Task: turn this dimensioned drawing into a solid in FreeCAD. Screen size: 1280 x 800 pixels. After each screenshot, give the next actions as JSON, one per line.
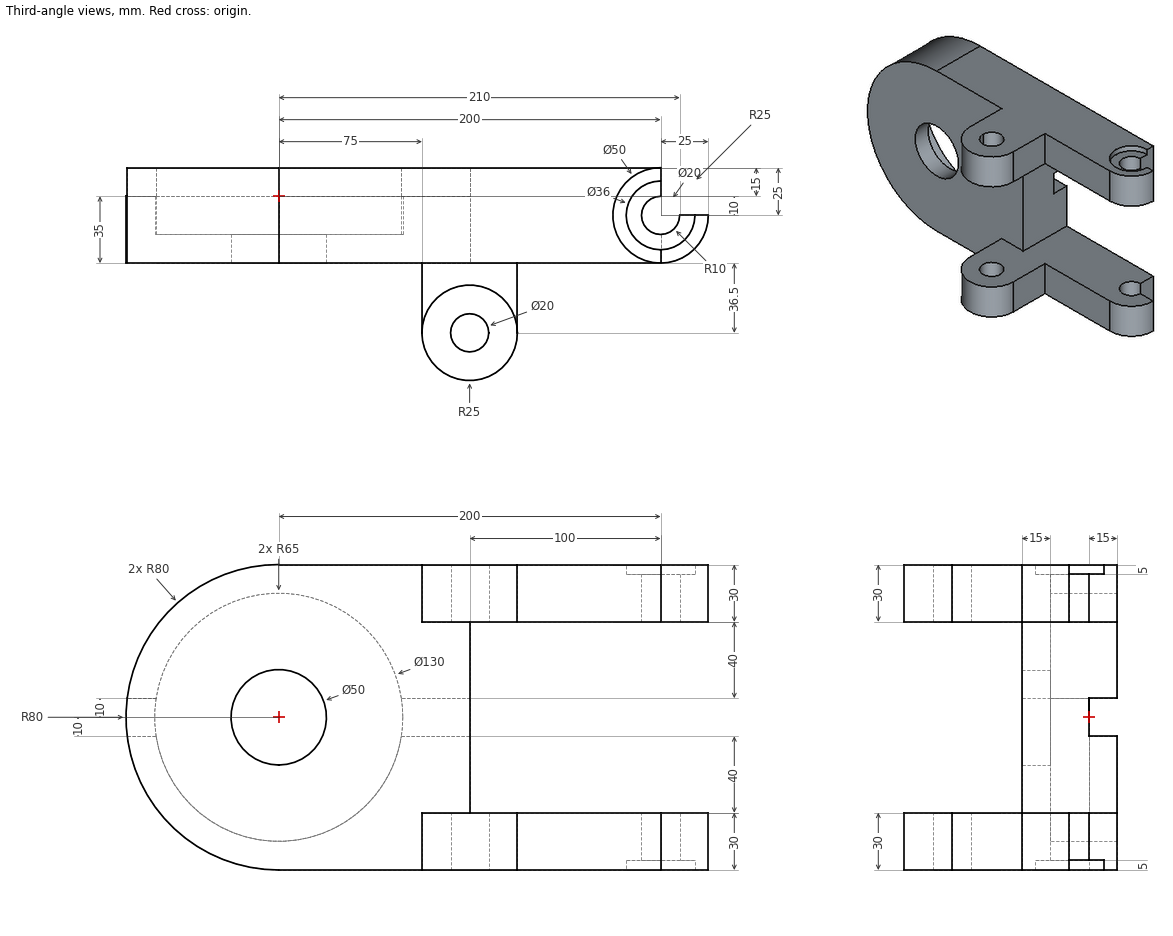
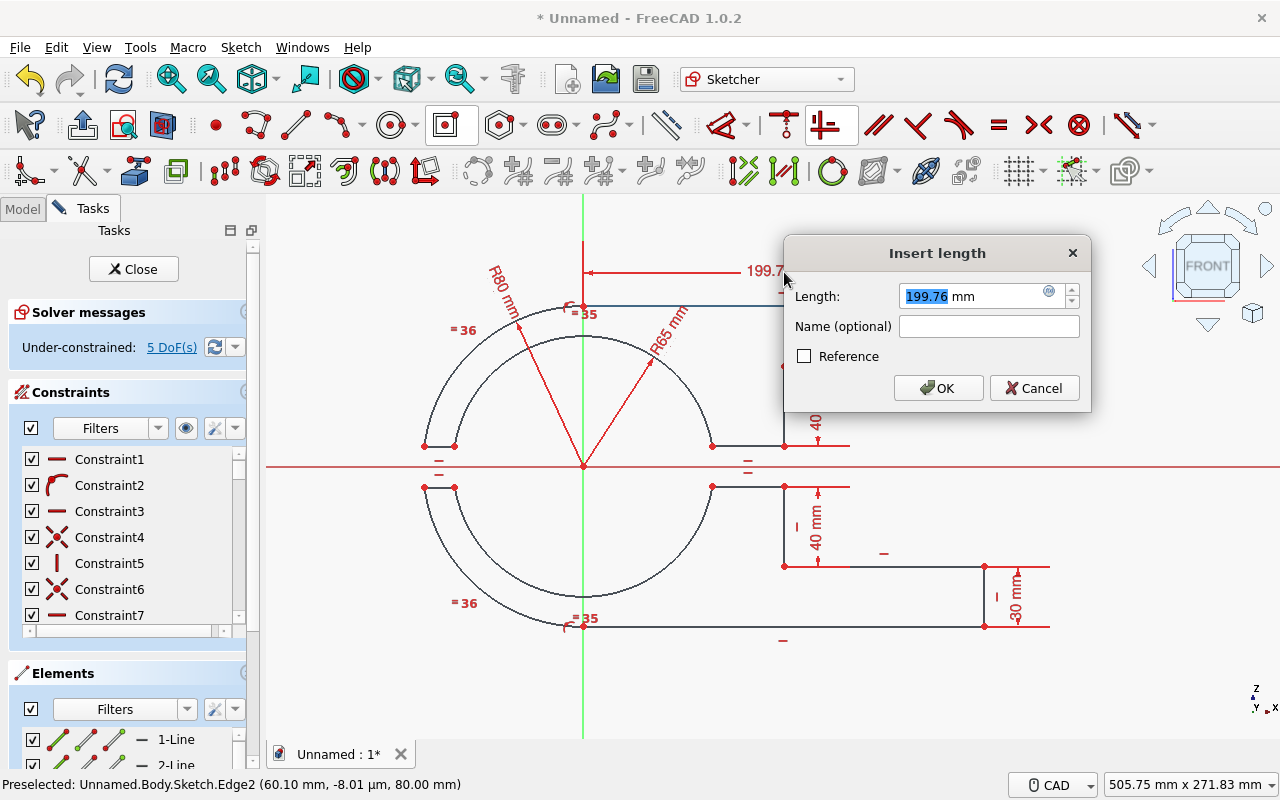
{"action": "type", "text": "200"}
{"action": "key", "text": "Return"}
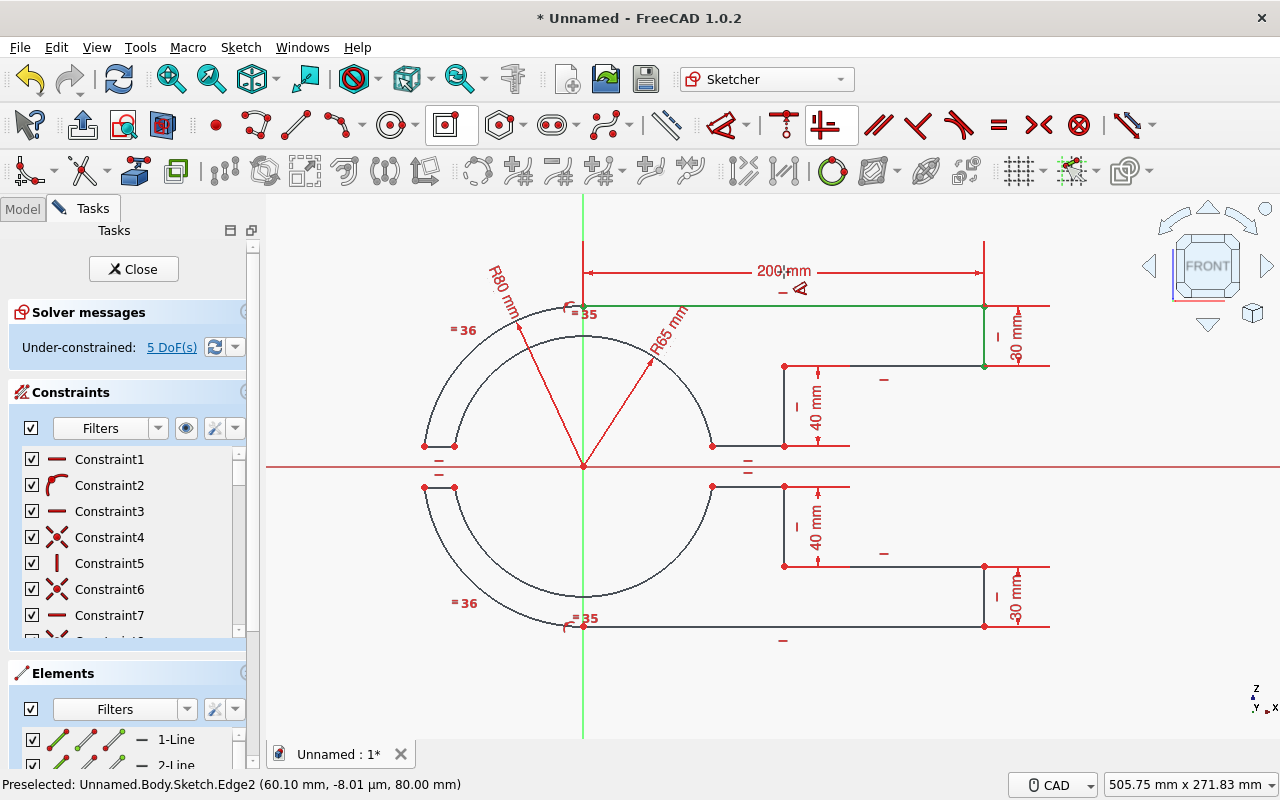
{"action": "left_click", "coordinate": [924, 366]}
{"action": "left_click", "coordinate": [884, 332]}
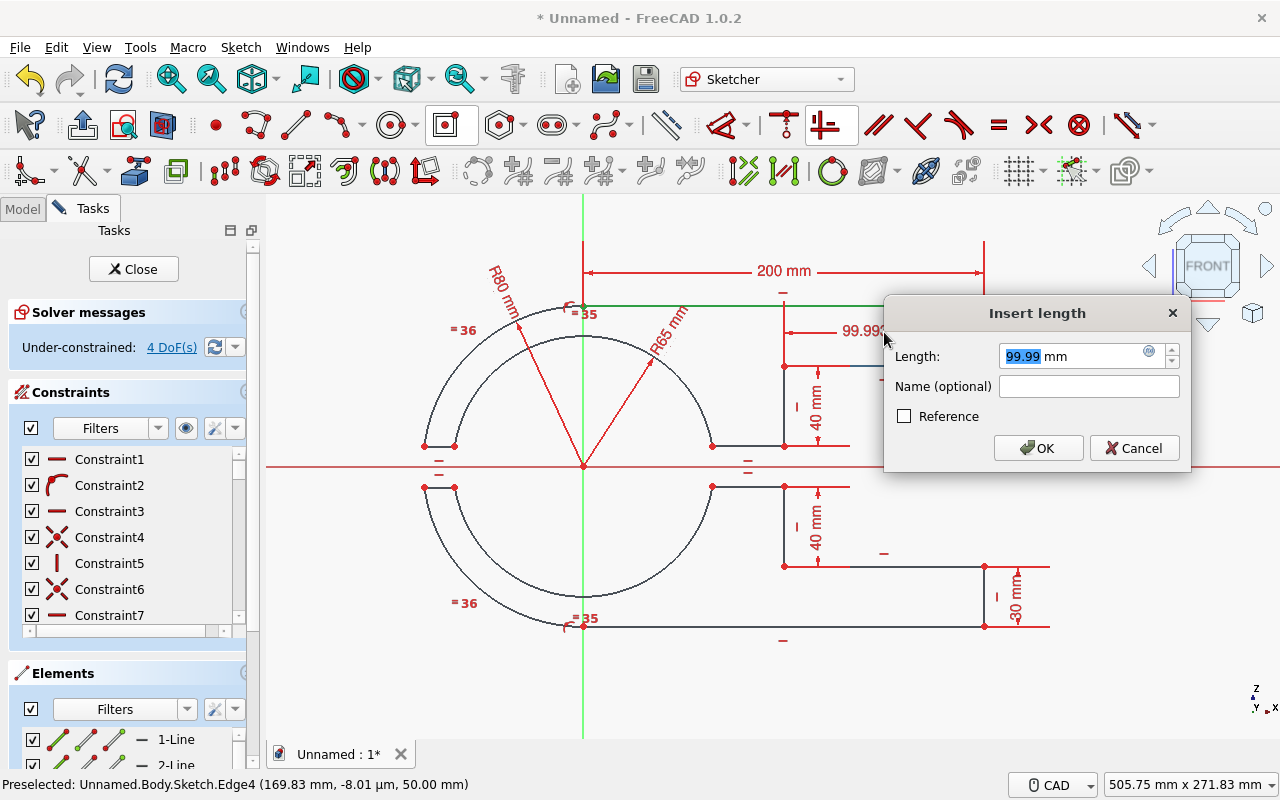
{"action": "type", "text": "100"}
{"action": "key", "text": "Return"}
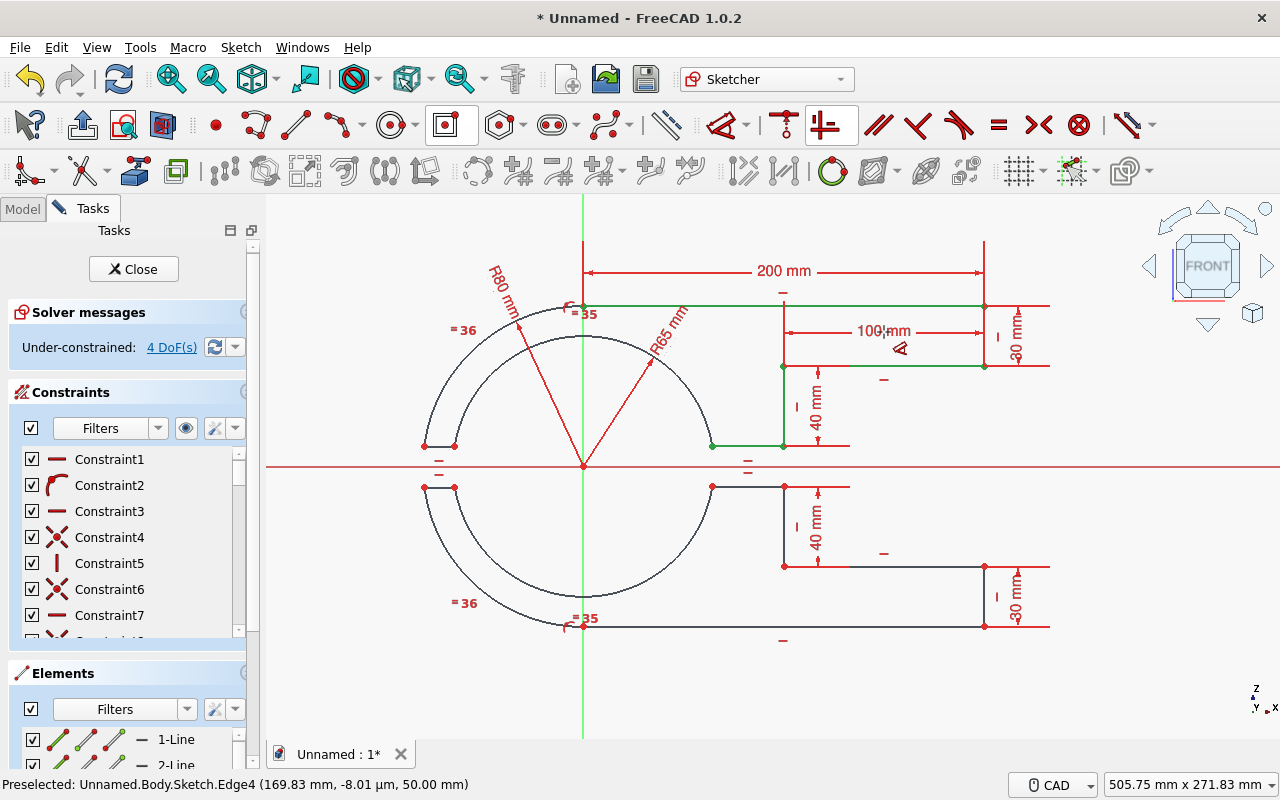
{"action": "left_click", "coordinate": [844, 567]}
{"action": "left_click", "coordinate": [884, 601]}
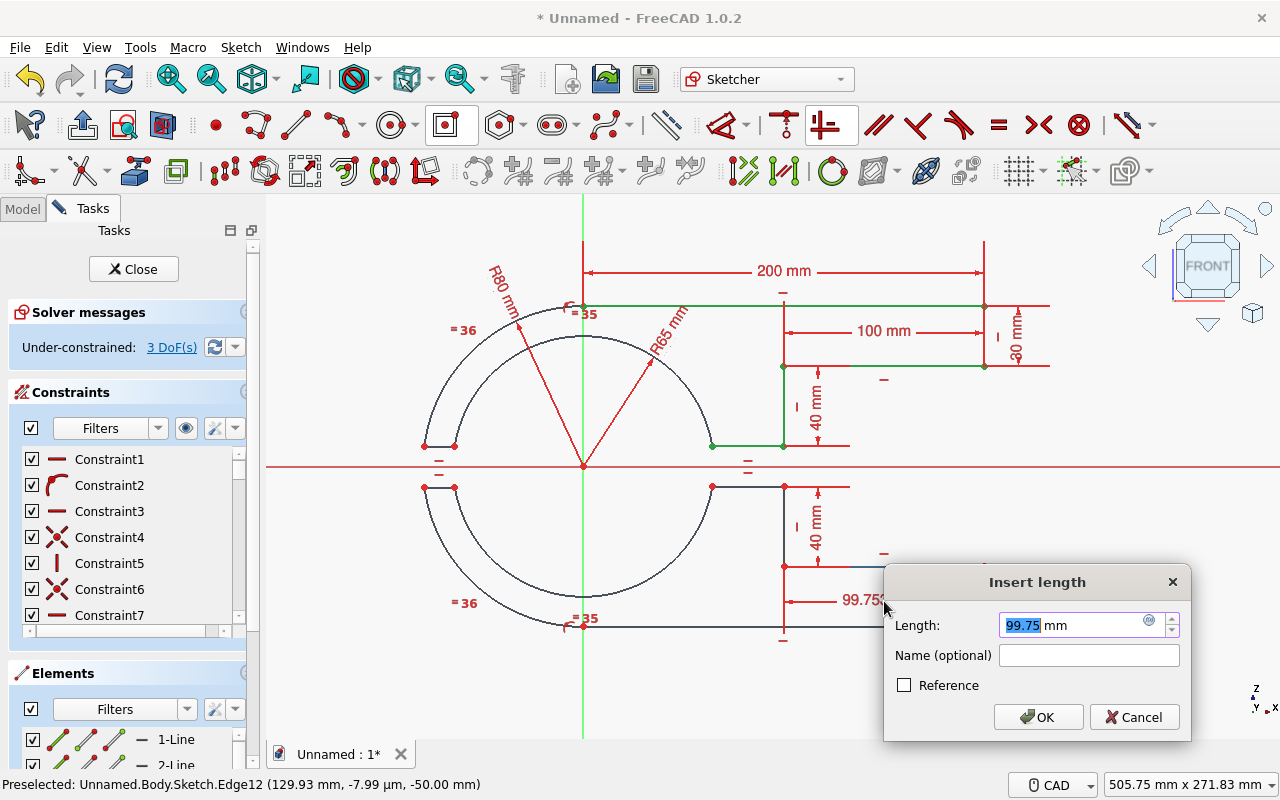
{"action": "type", "text": "100"}
{"action": "key", "text": "Return"}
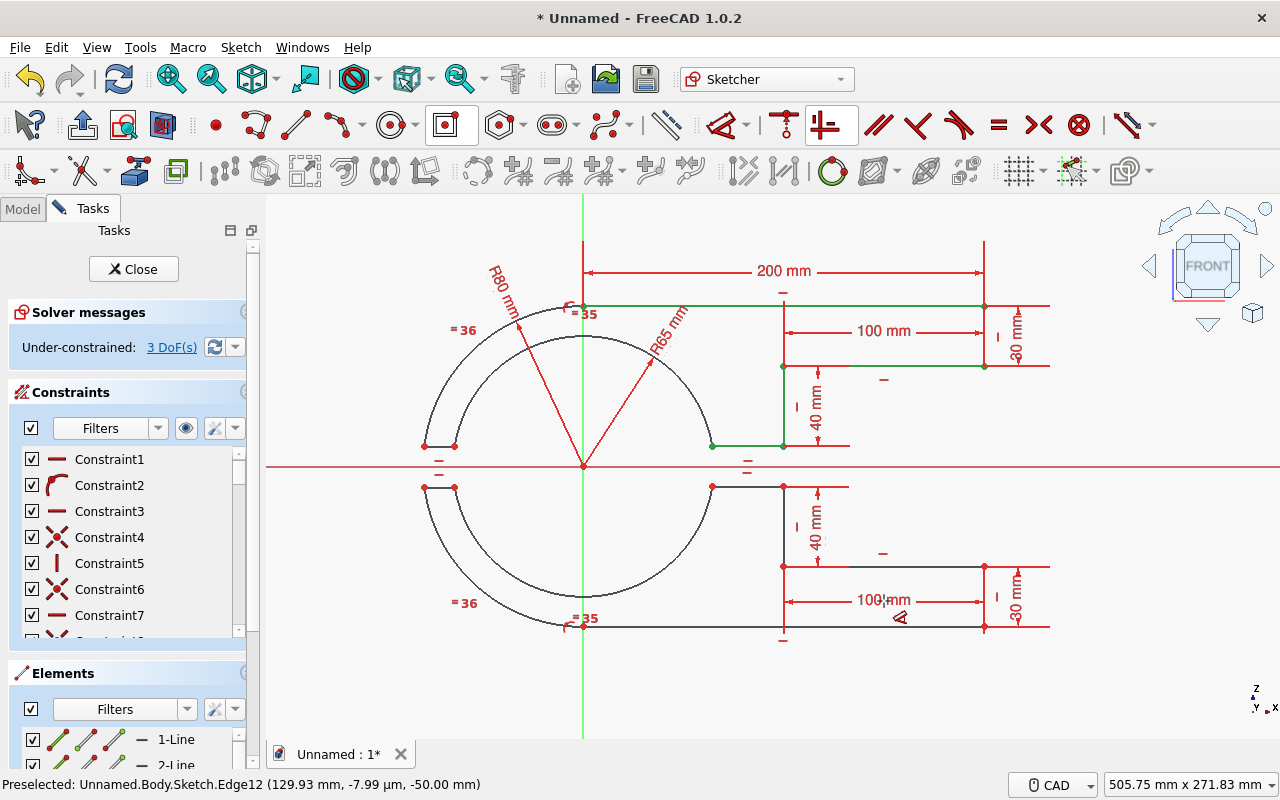
{"action": "left_click", "coordinate": [864, 627]}
{"action": "left_click", "coordinate": [784, 661]}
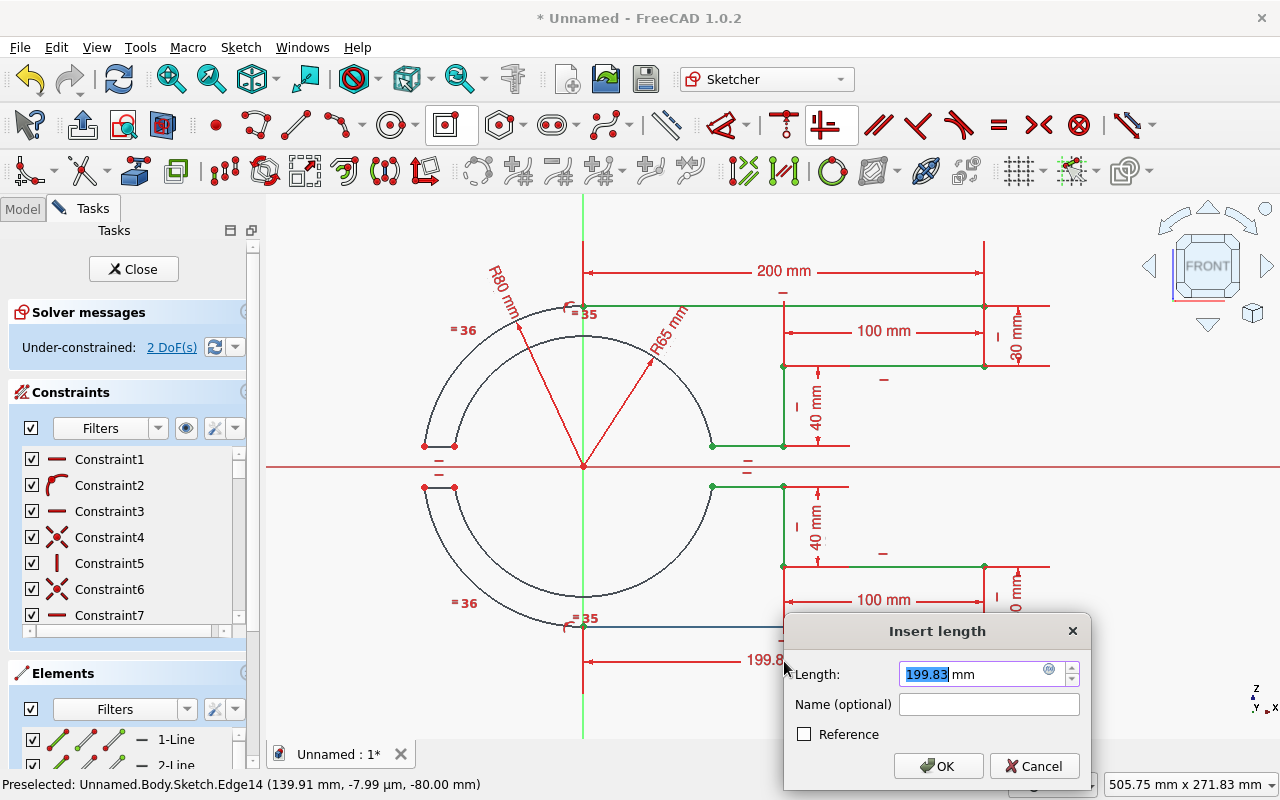
{"action": "type", "text": "200"}
{"action": "key", "text": "Return"}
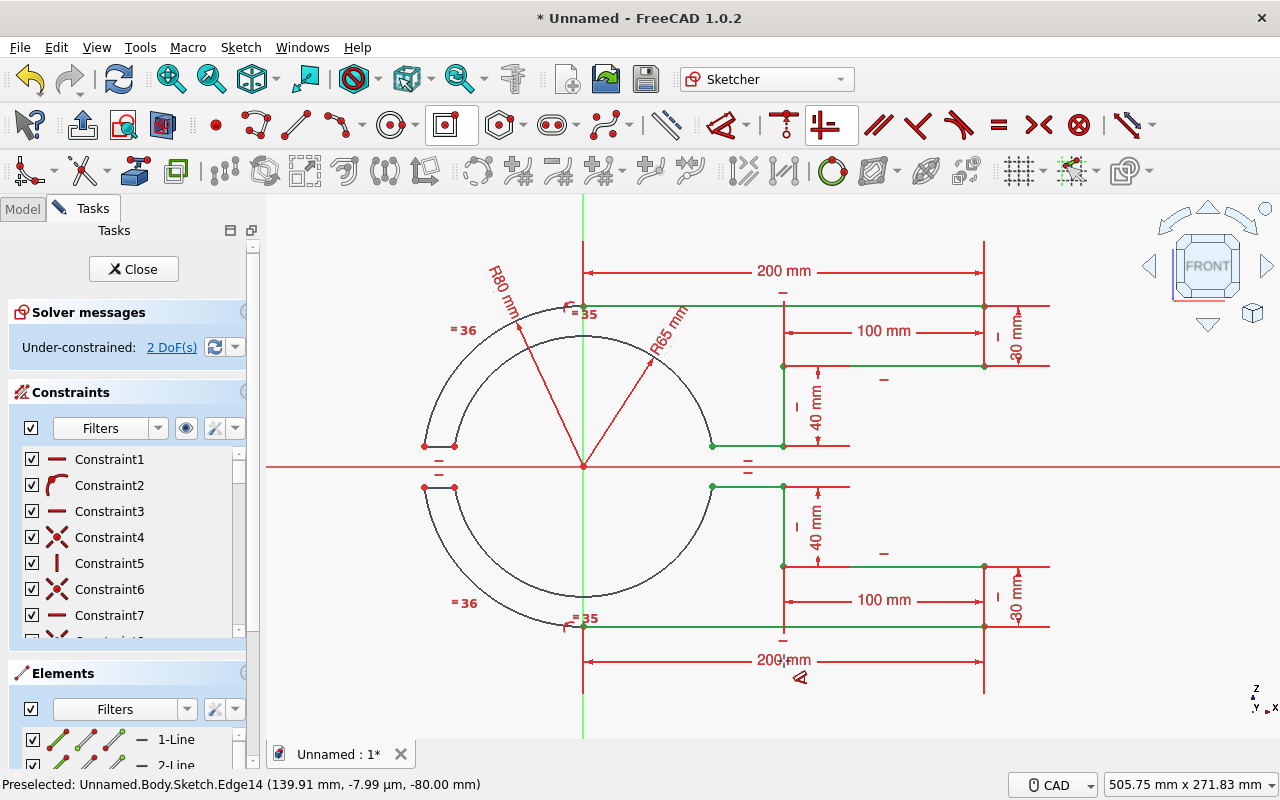
{"action": "scroll", "coordinate": [455, 447], "scroll_direction": "up", "scroll_amount": 4}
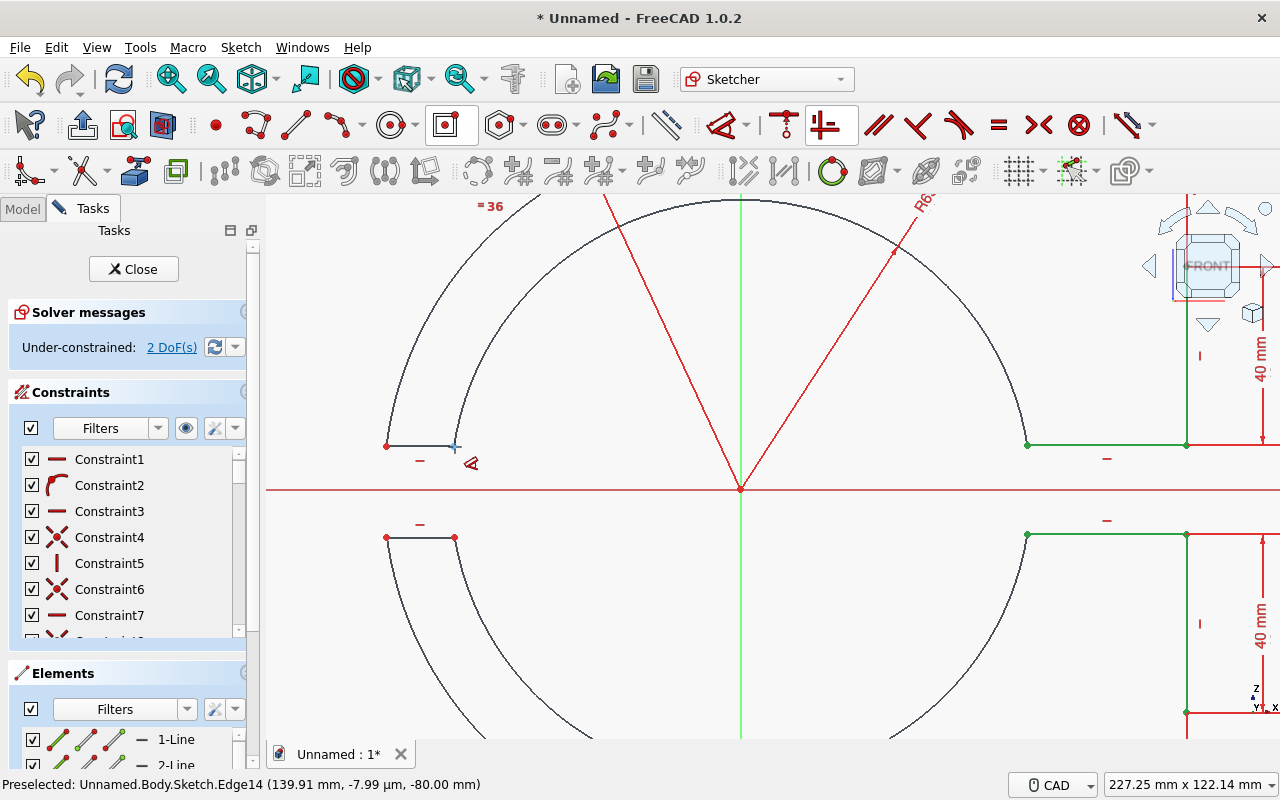
{"action": "left_click", "coordinate": [454, 446]}
{"action": "left_click", "coordinate": [420, 468]}